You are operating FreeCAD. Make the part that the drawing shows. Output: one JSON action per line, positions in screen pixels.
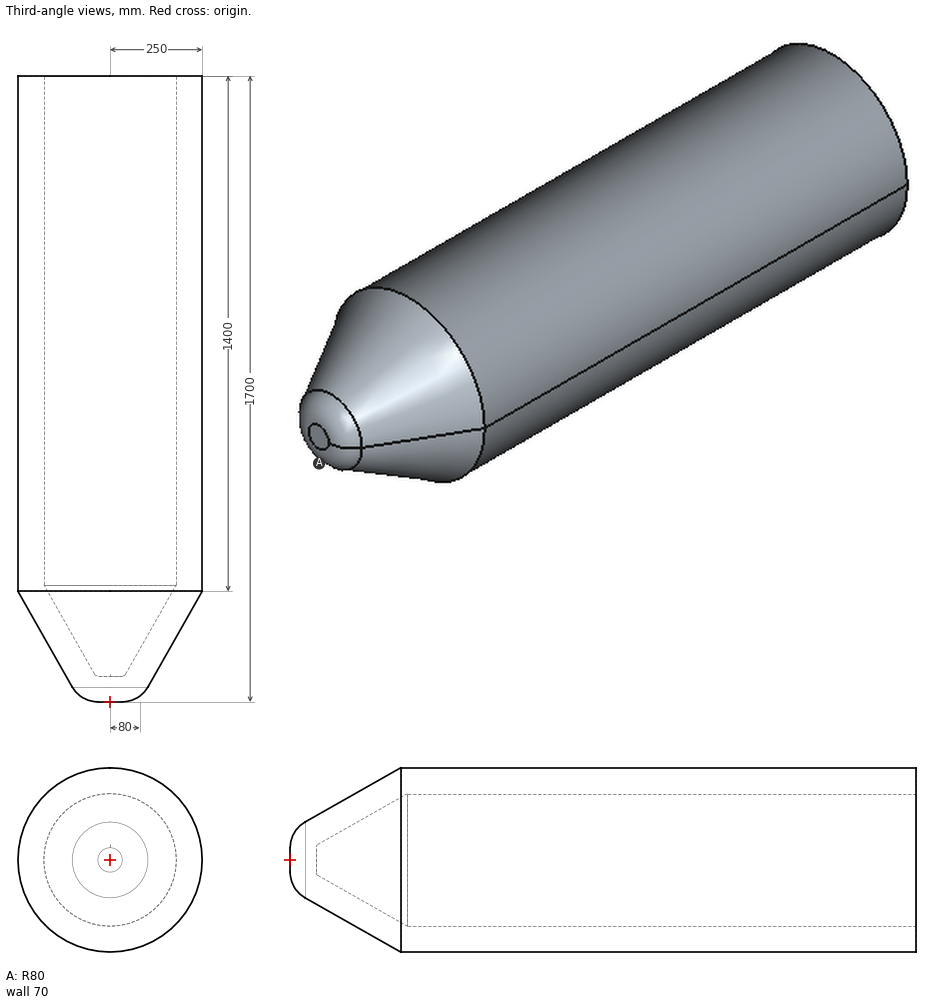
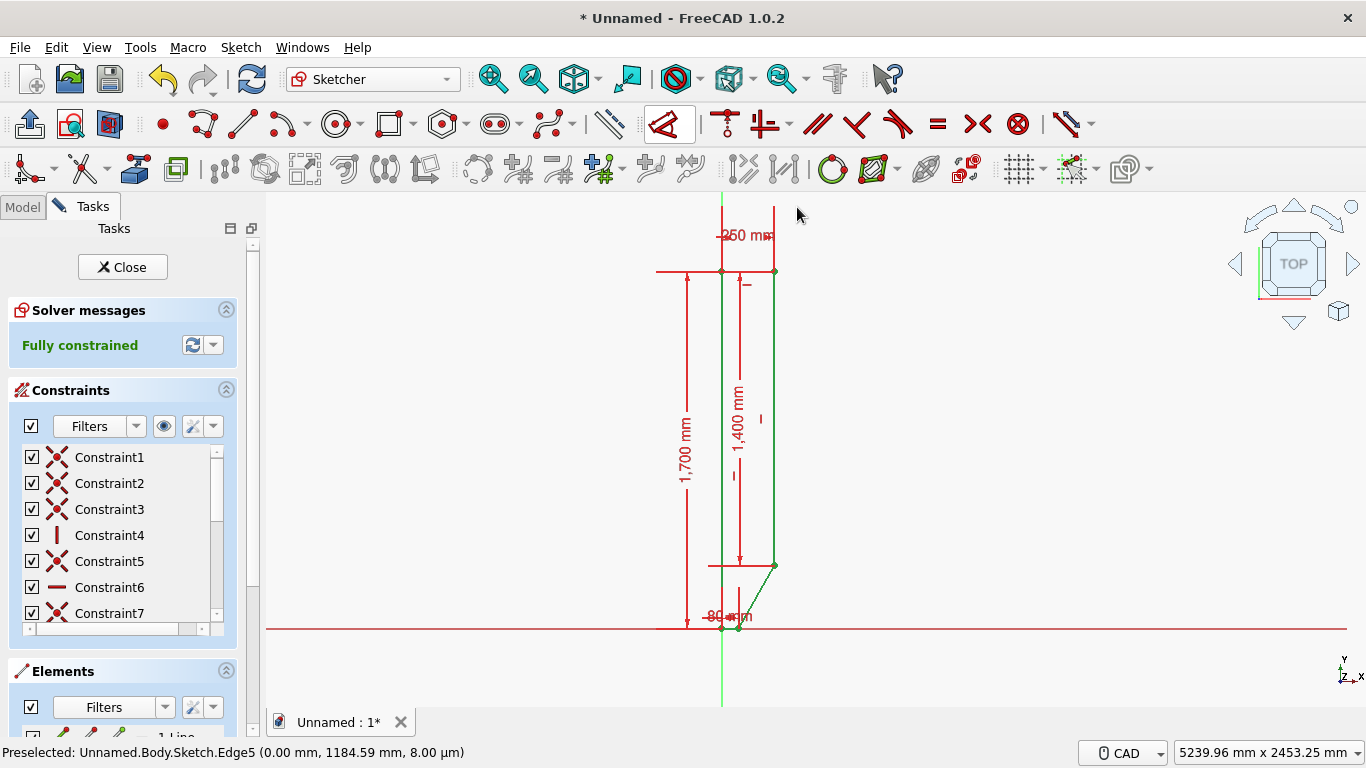
{"action": "left_click", "coordinate": [123, 267]}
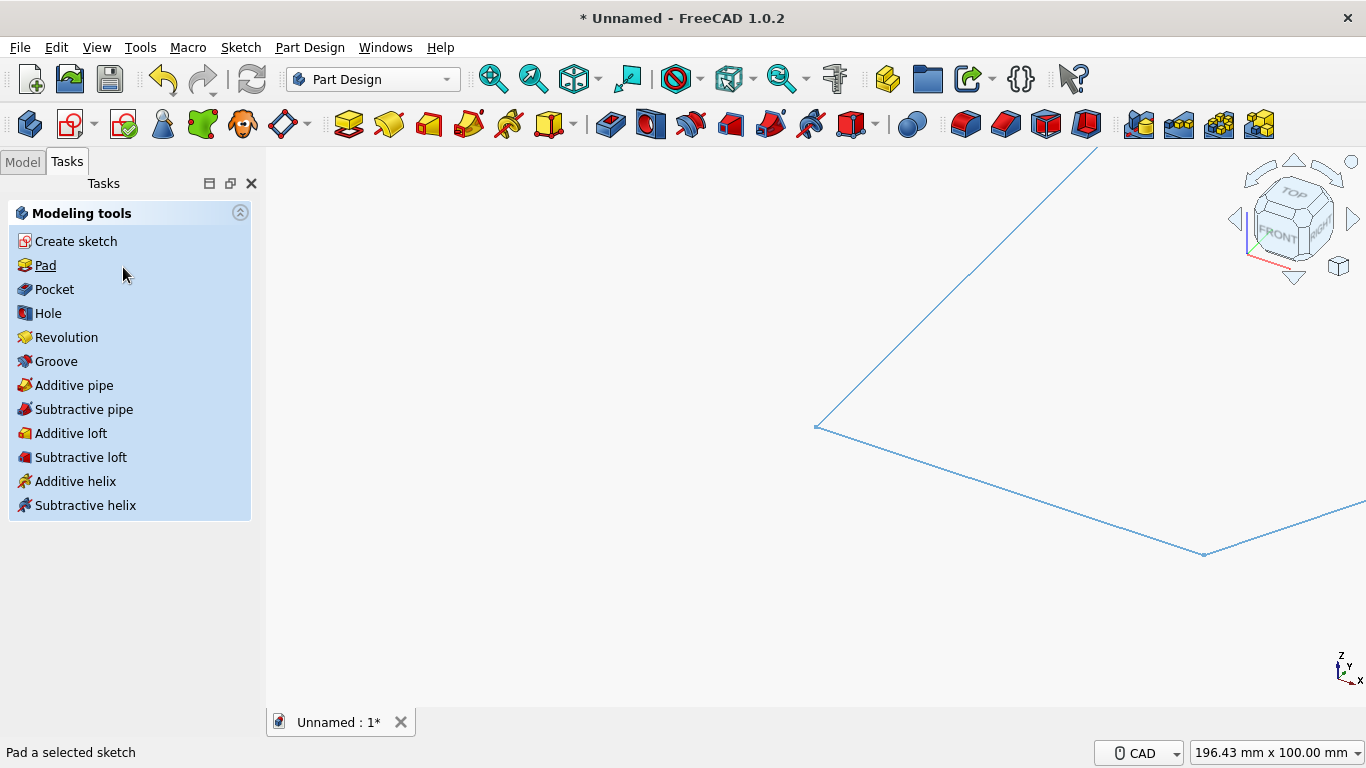
{"action": "left_click", "coordinate": [390, 124]}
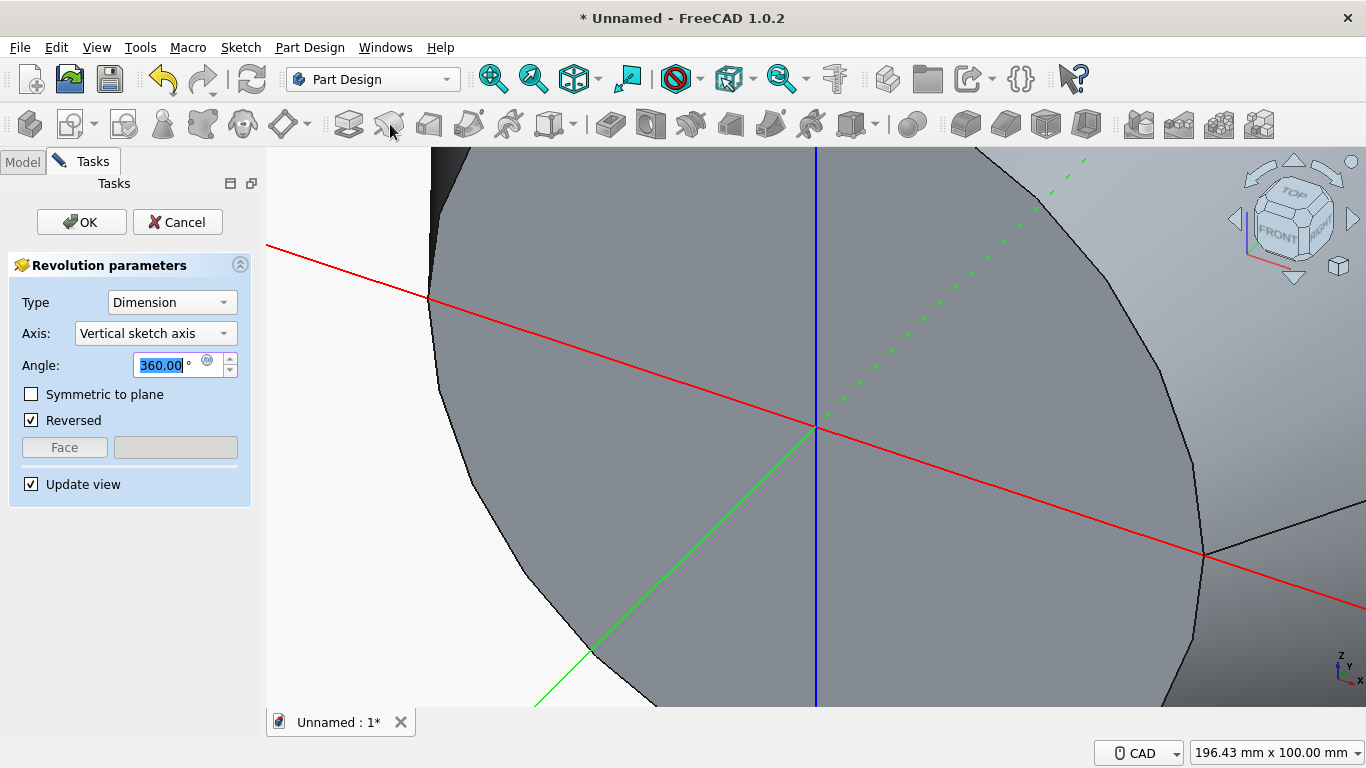
{"action": "left_click", "coordinate": [82, 222]}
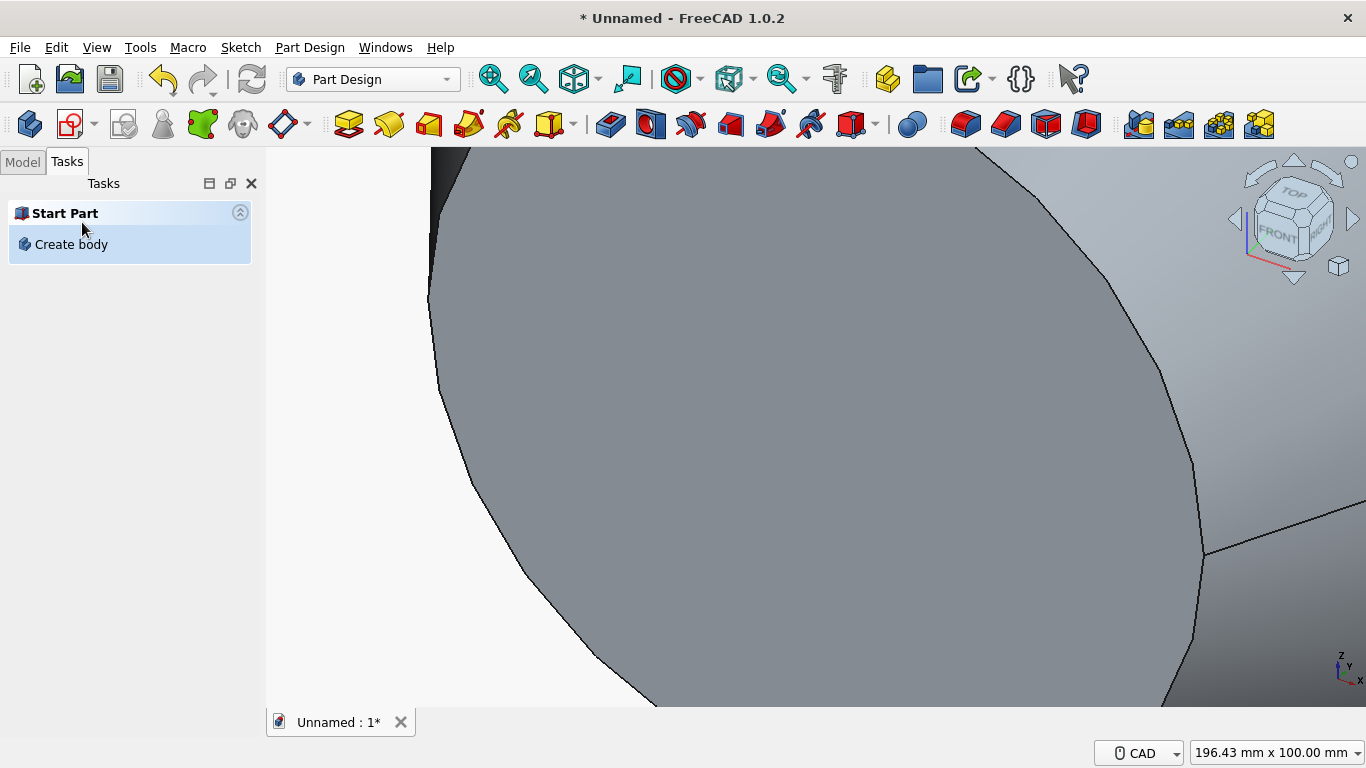
{"action": "left_click", "coordinate": [494, 80]}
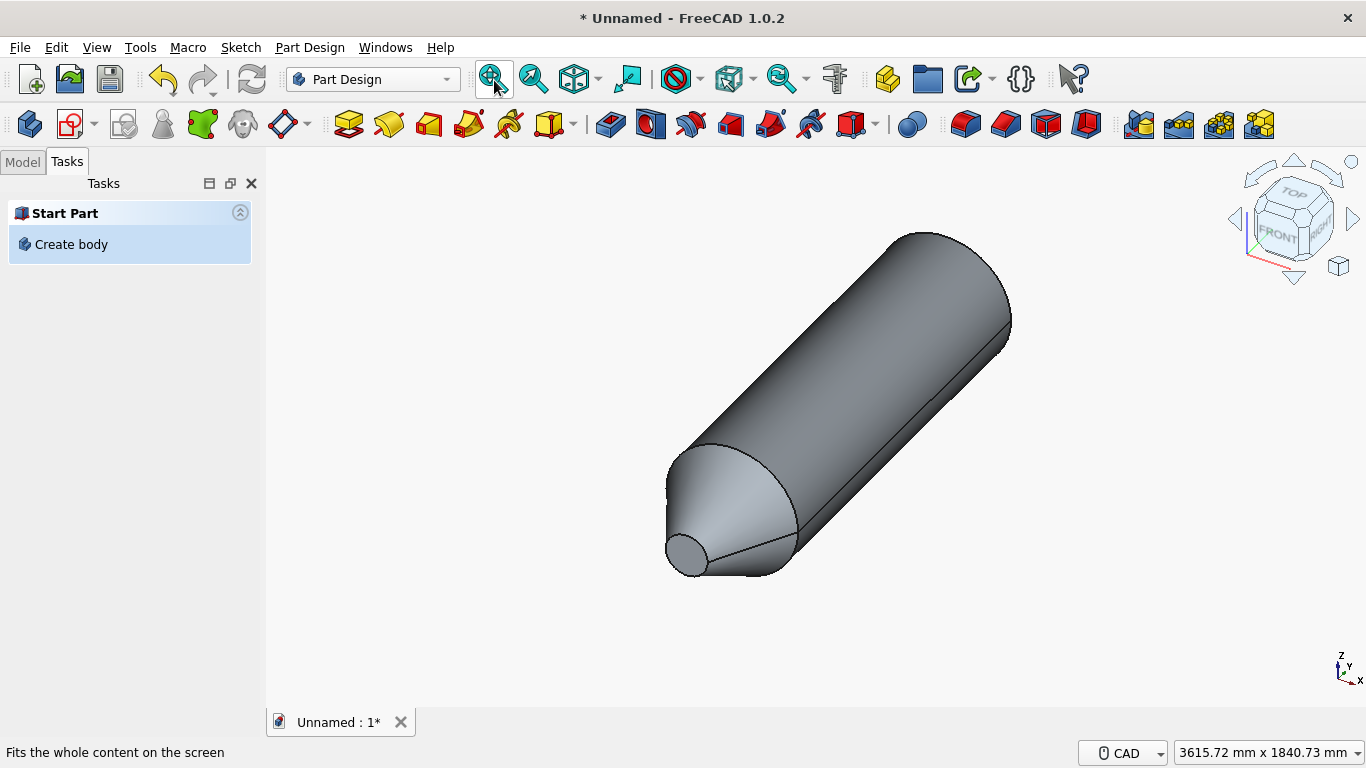
{"action": "left_click", "coordinate": [670, 537]}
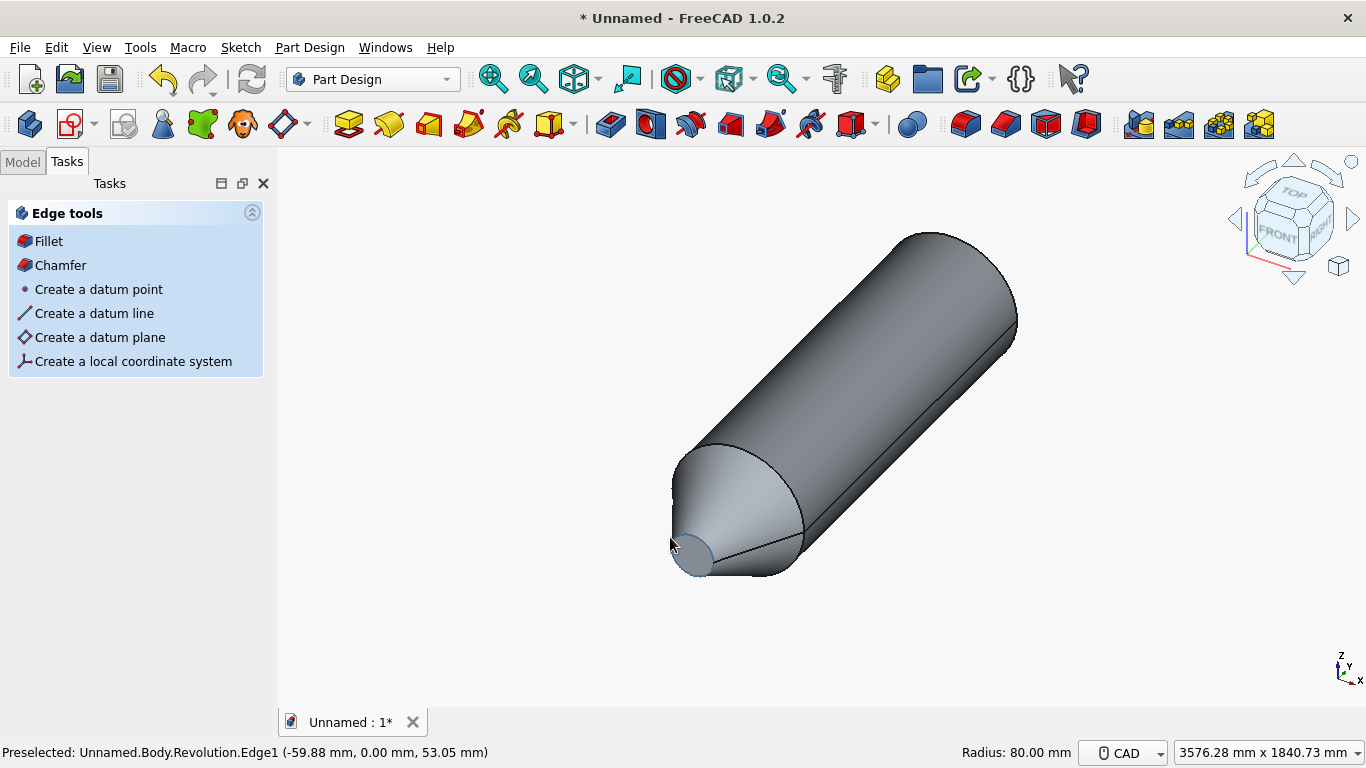
{"action": "left_click", "coordinate": [966, 124]}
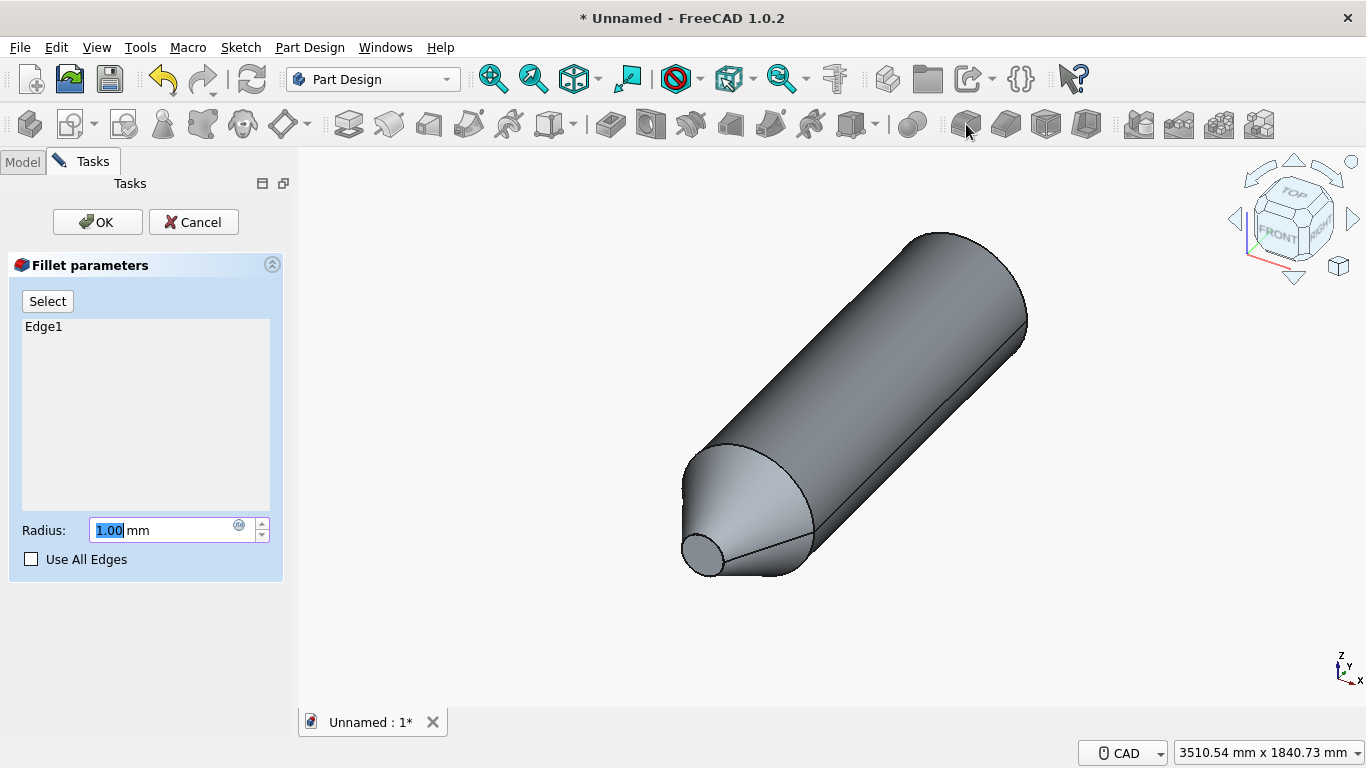
{"action": "type", "text": "80"}
{"action": "key", "text": "Tab"}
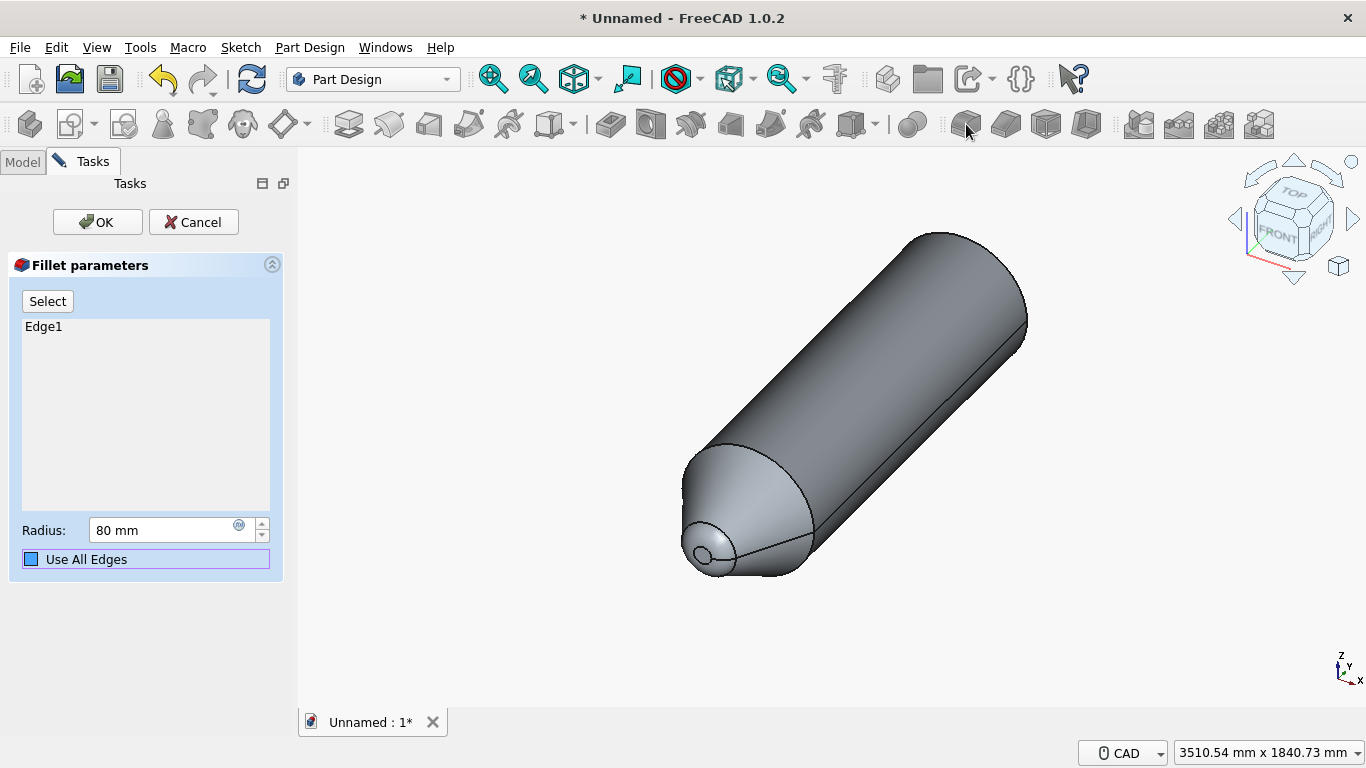
{"action": "left_click", "coordinate": [98, 222]}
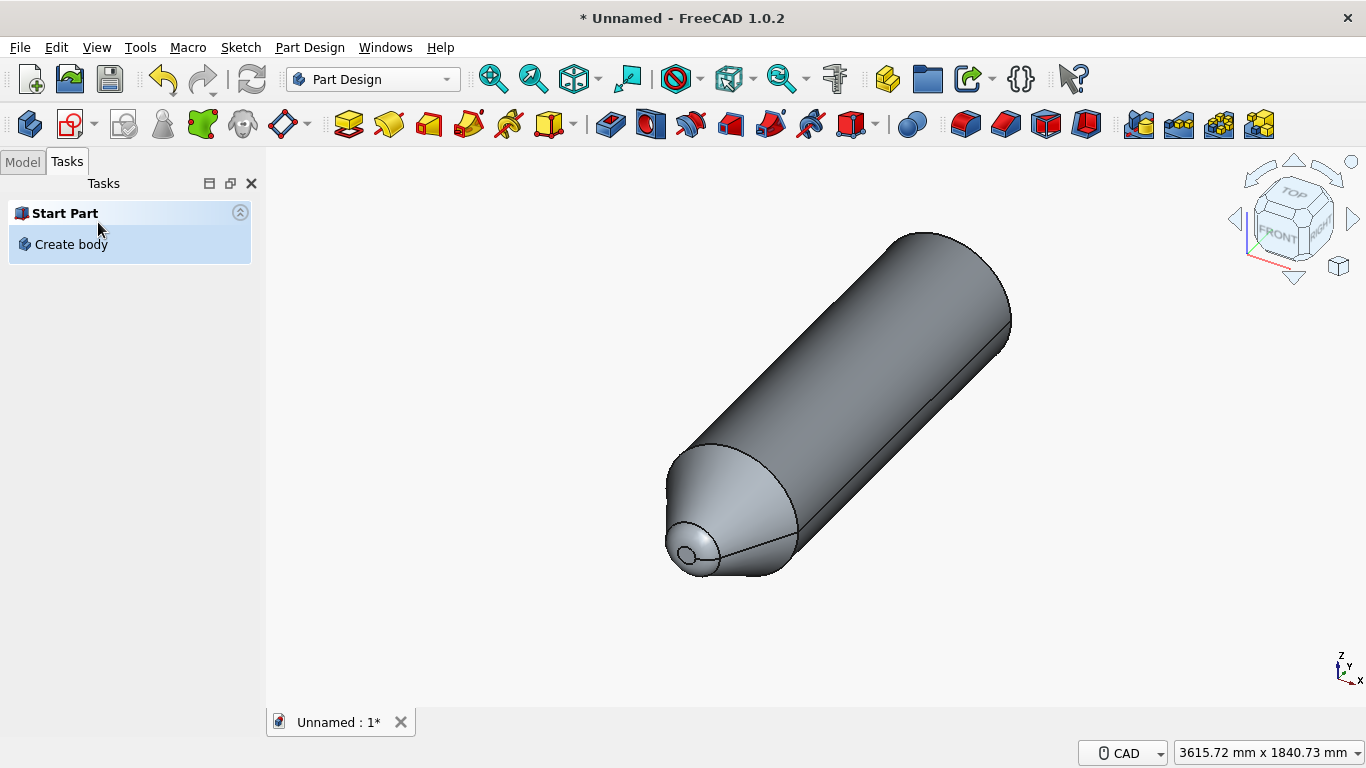
{"action": "key", "text": "0"}